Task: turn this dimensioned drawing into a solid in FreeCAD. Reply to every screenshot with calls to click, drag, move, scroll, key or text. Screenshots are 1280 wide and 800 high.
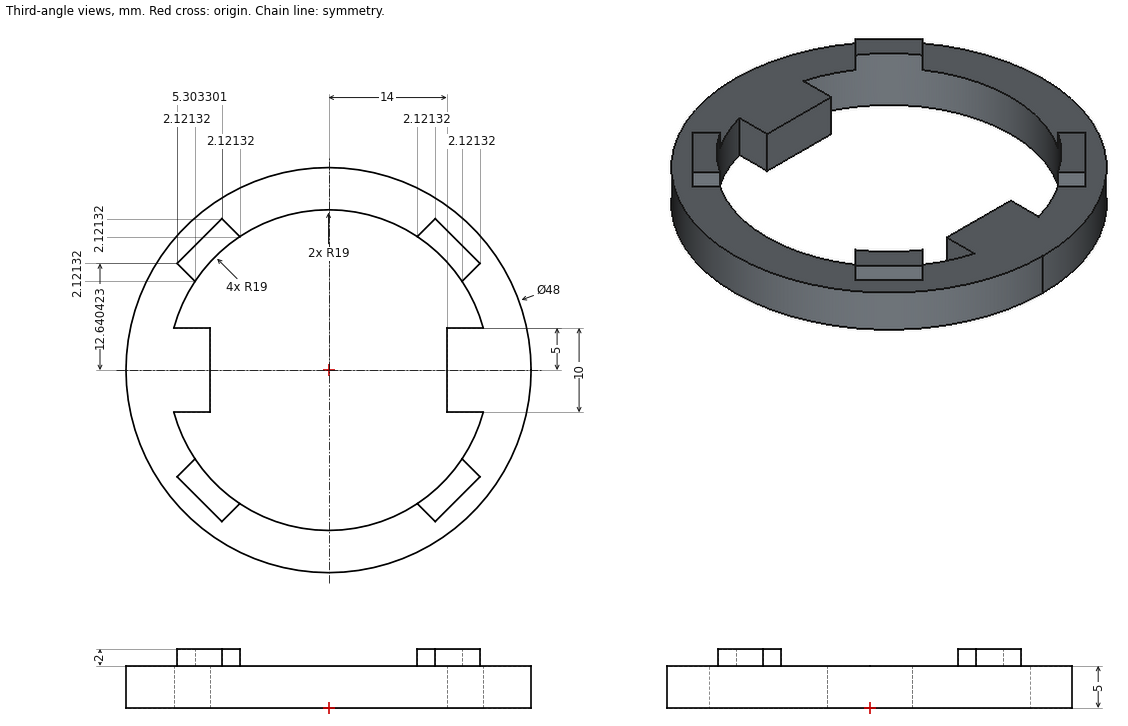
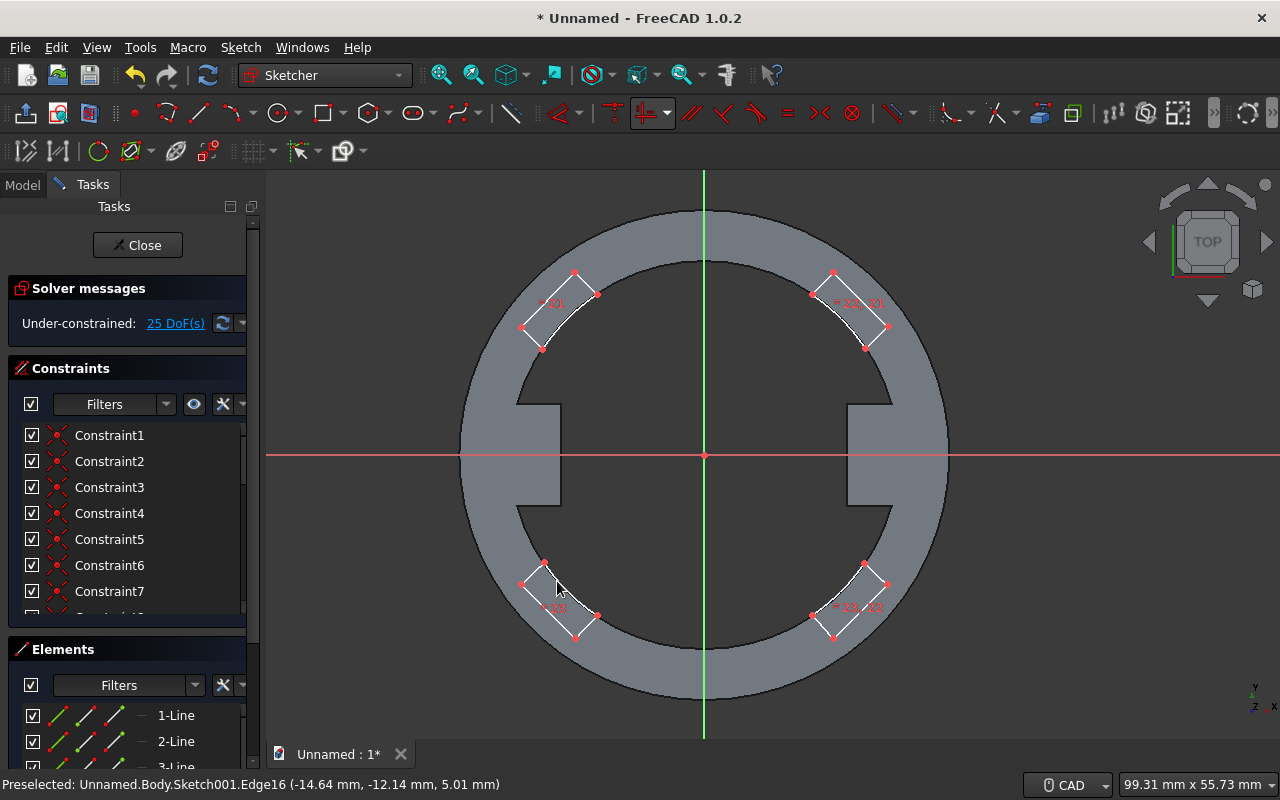
click(521, 327)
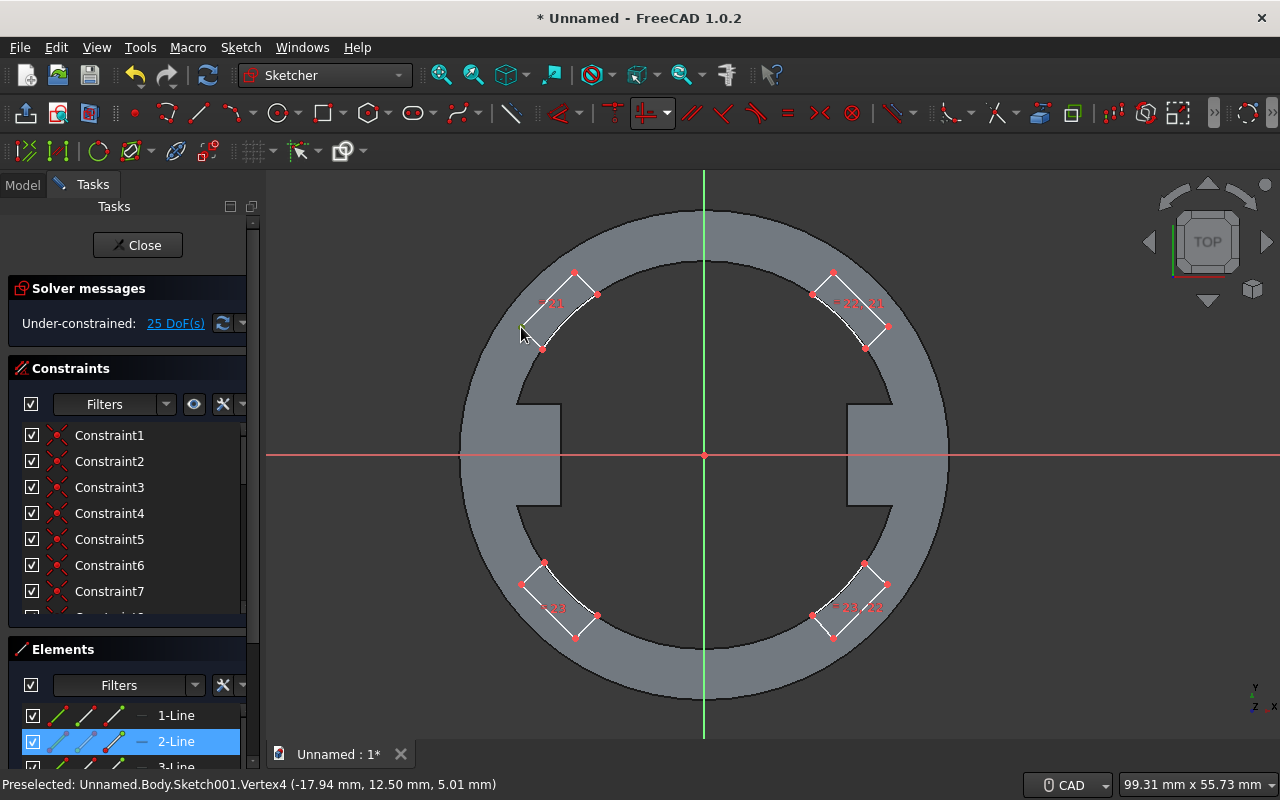
click(888, 327)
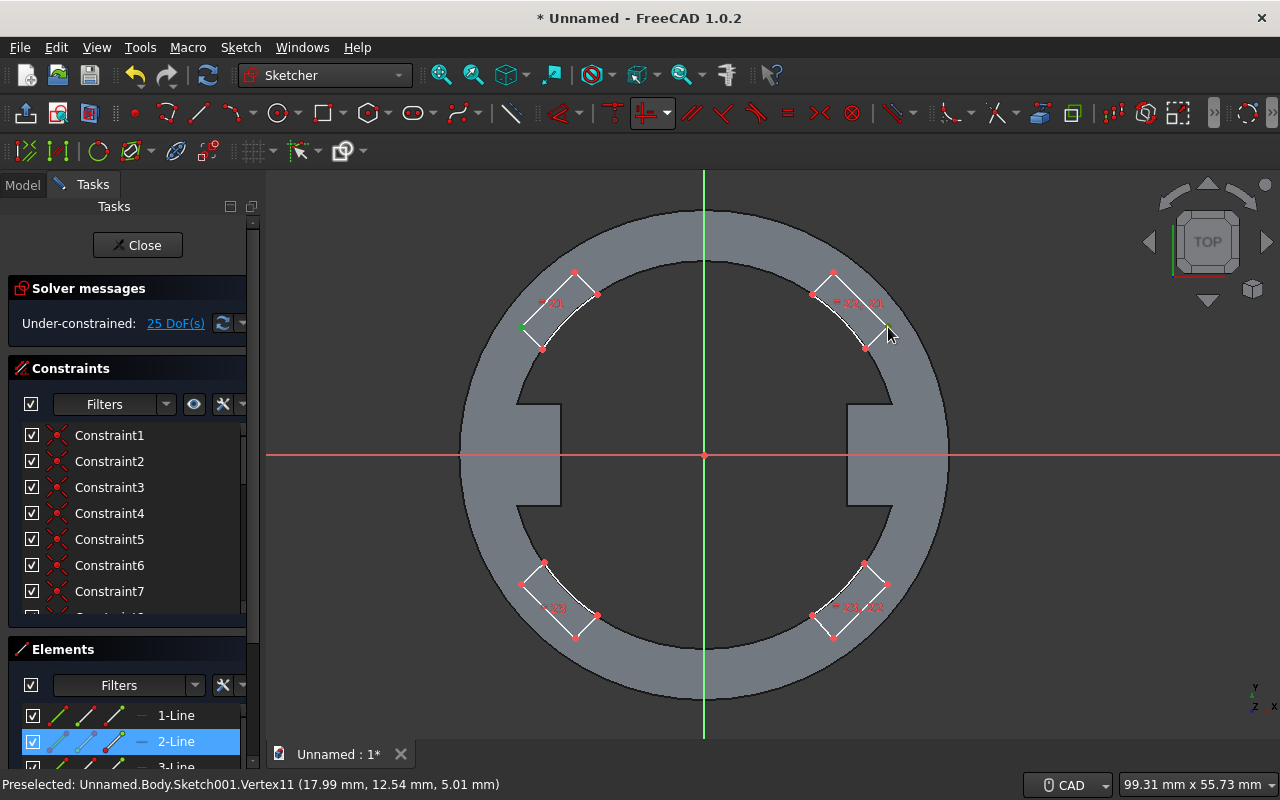
click(704, 674)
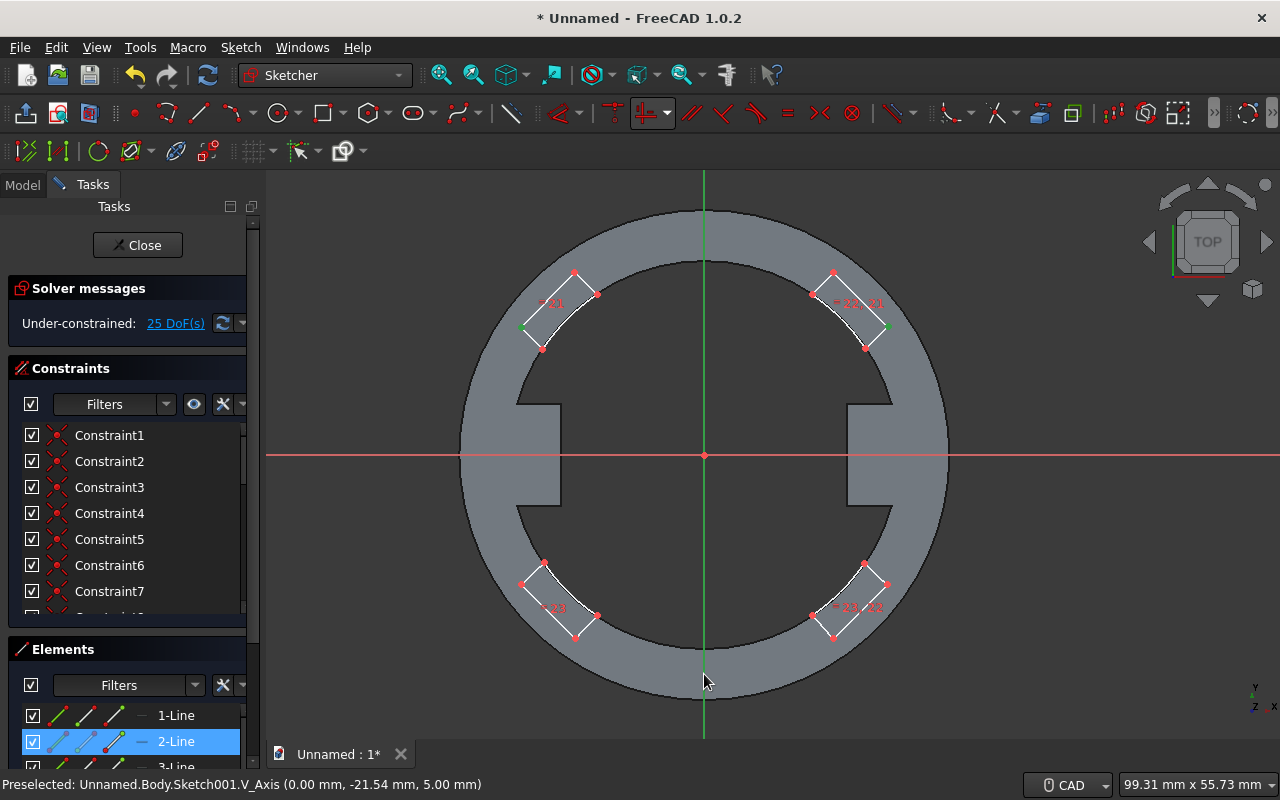
key(s)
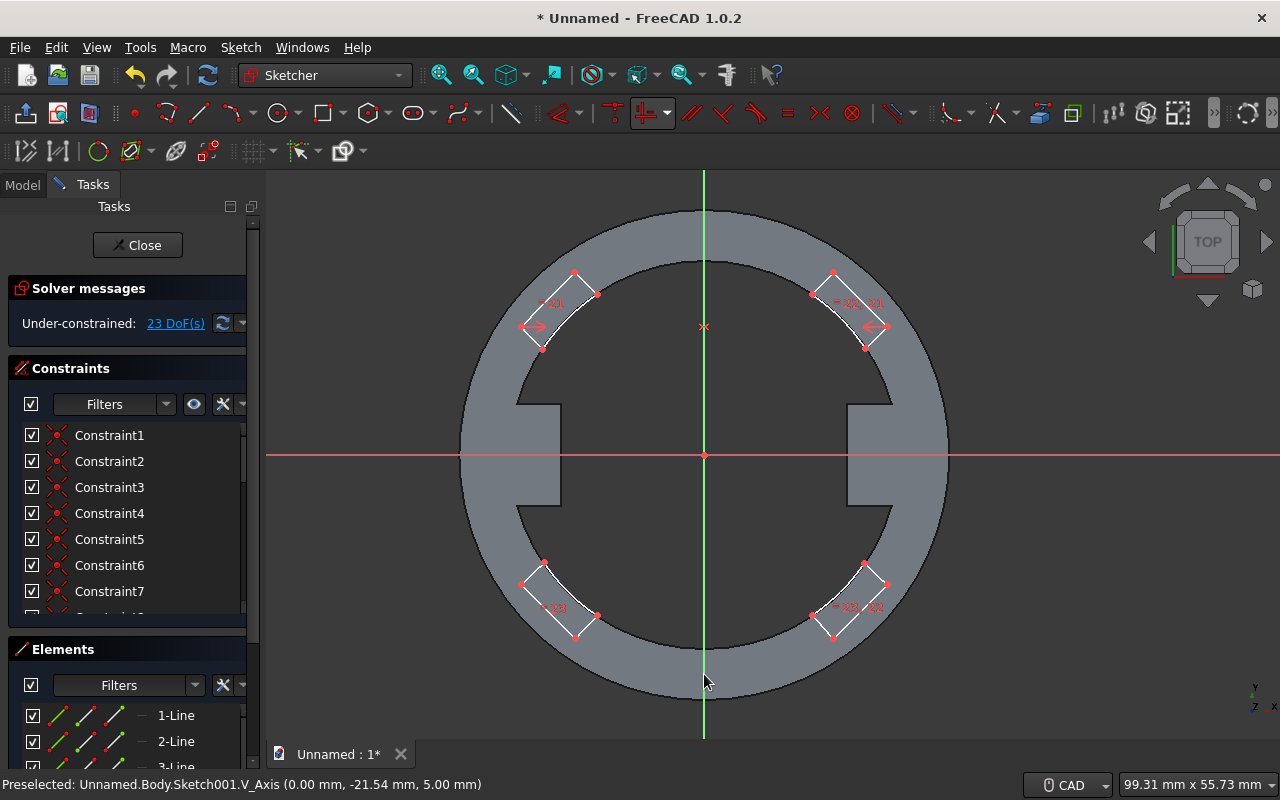
click(575, 272)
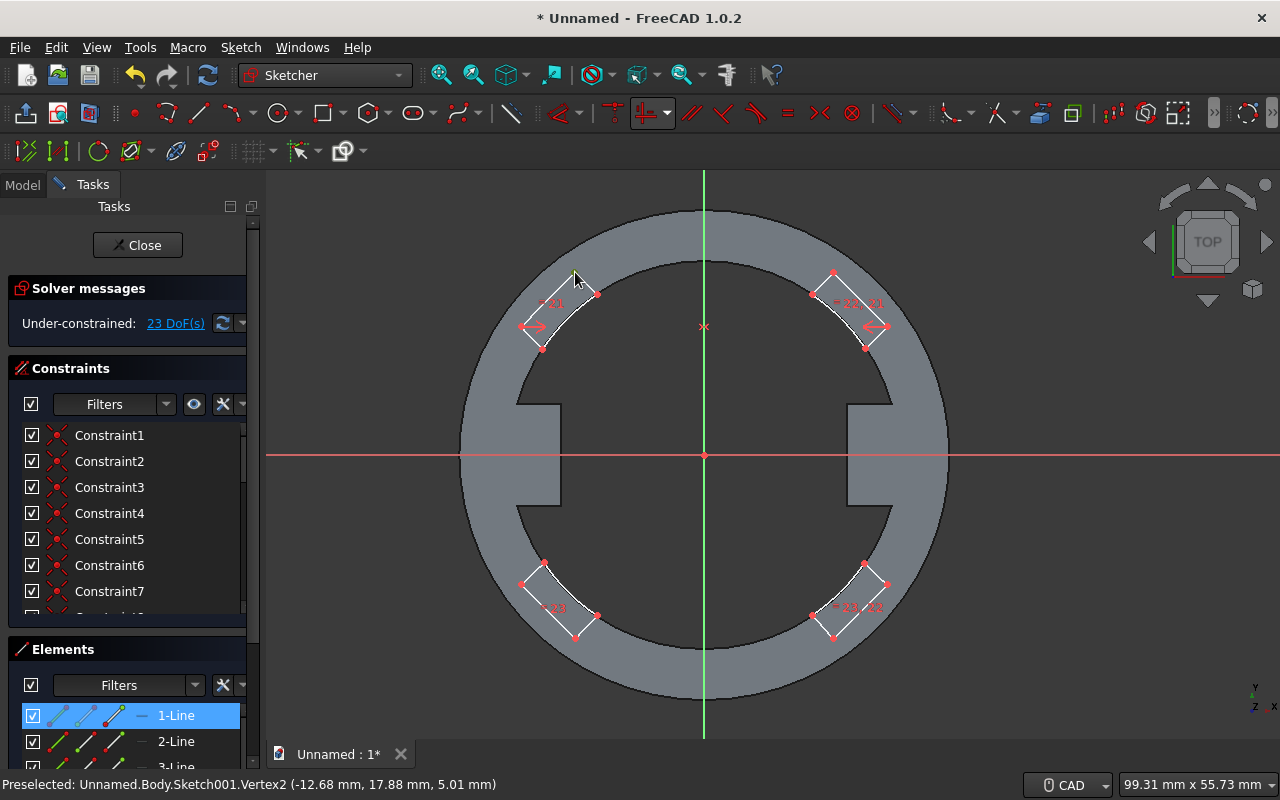
click(833, 273)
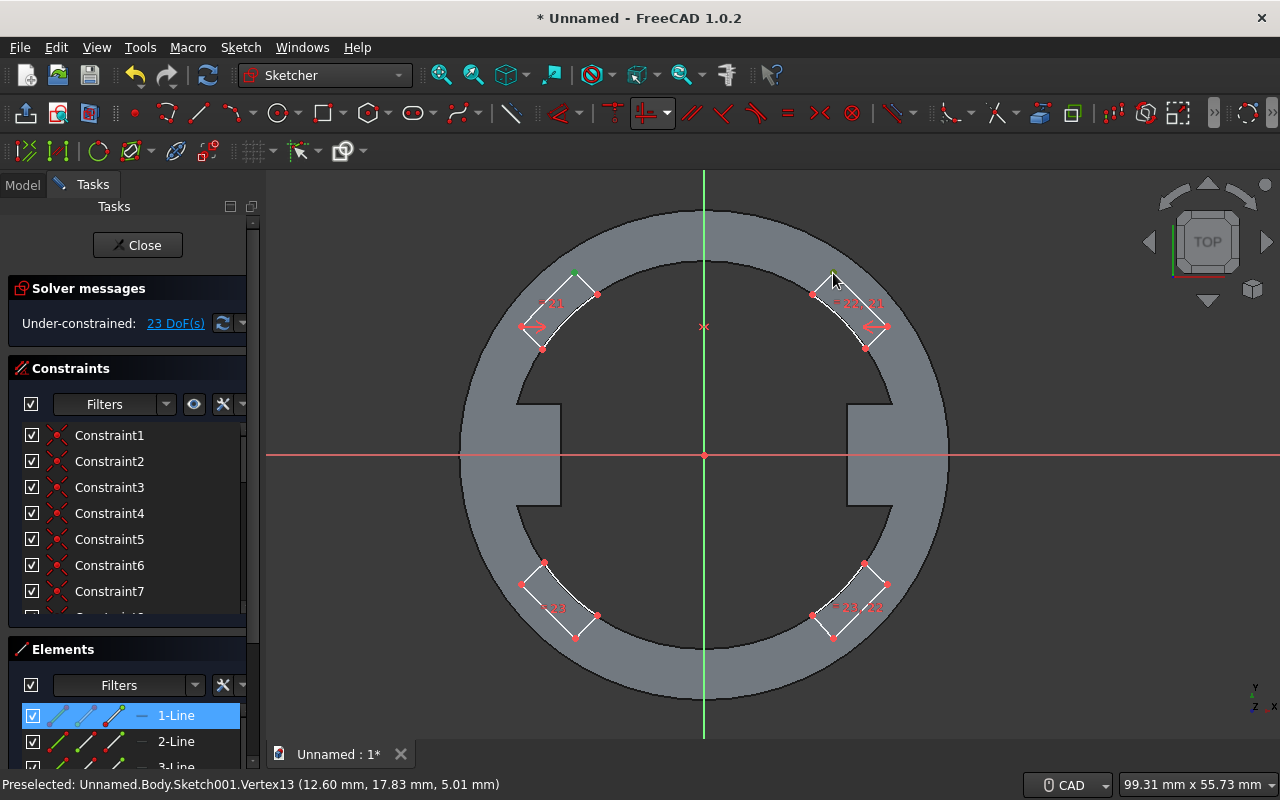
click(704, 674)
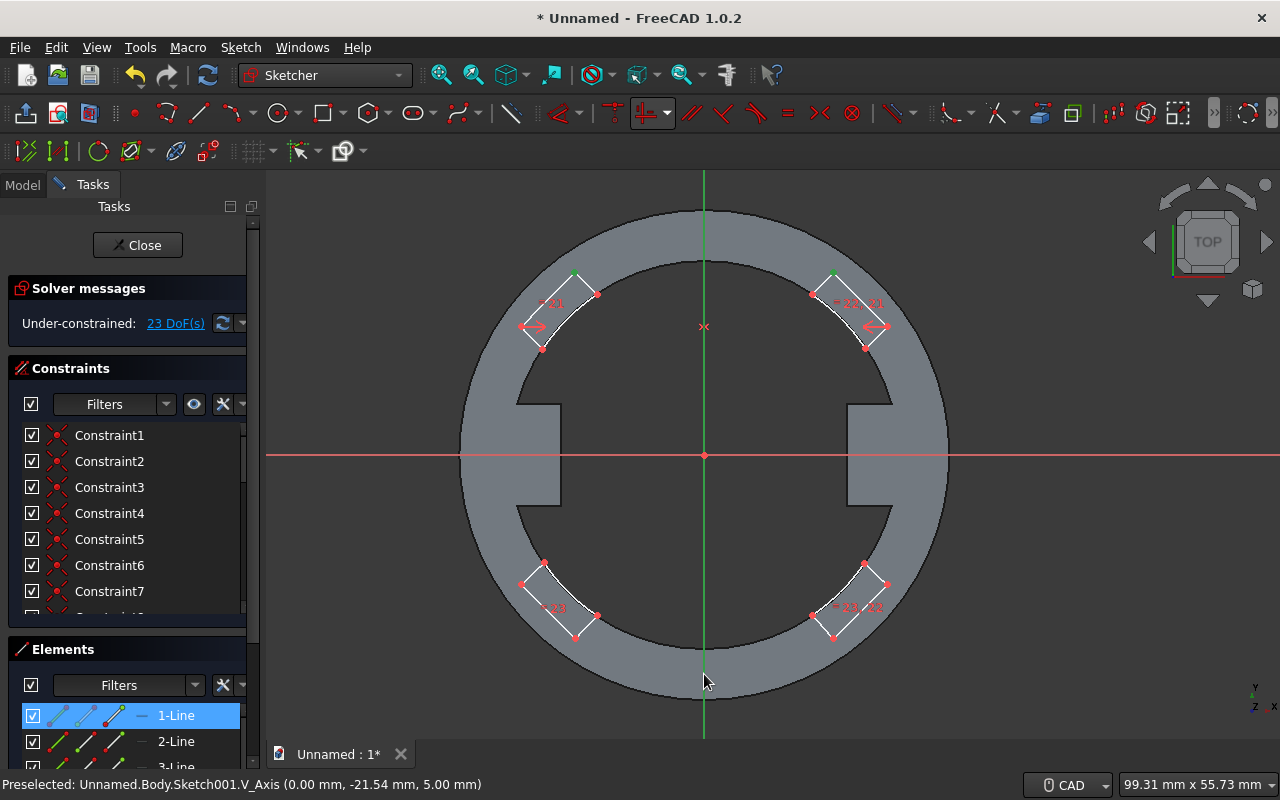
key(s)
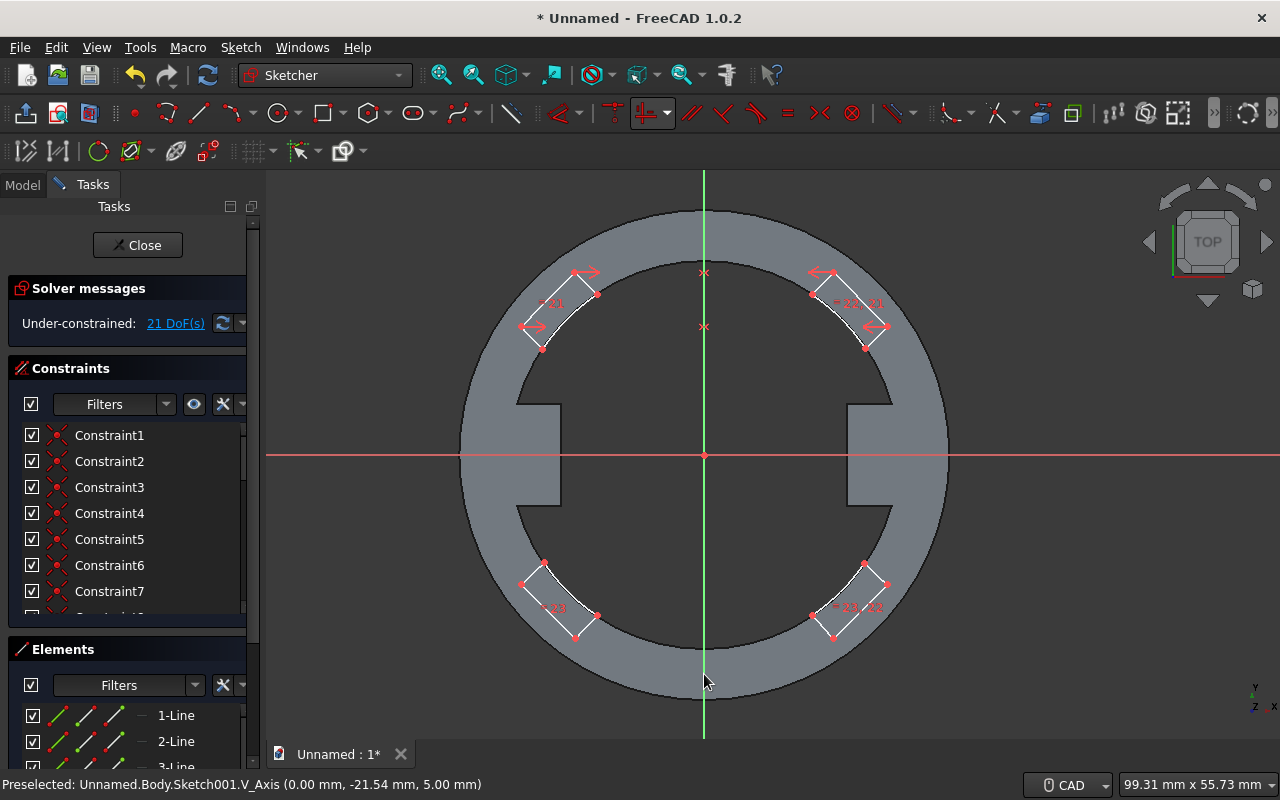
click(834, 272)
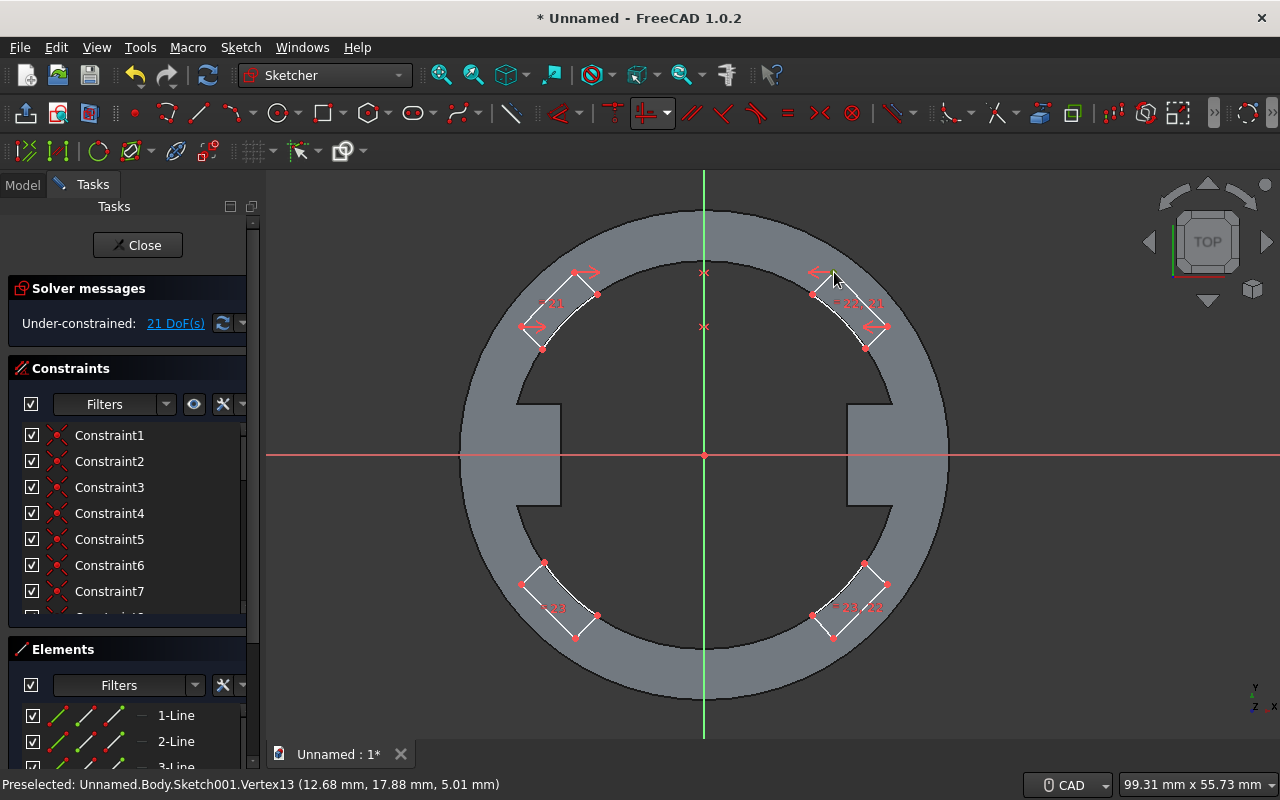
click(833, 639)